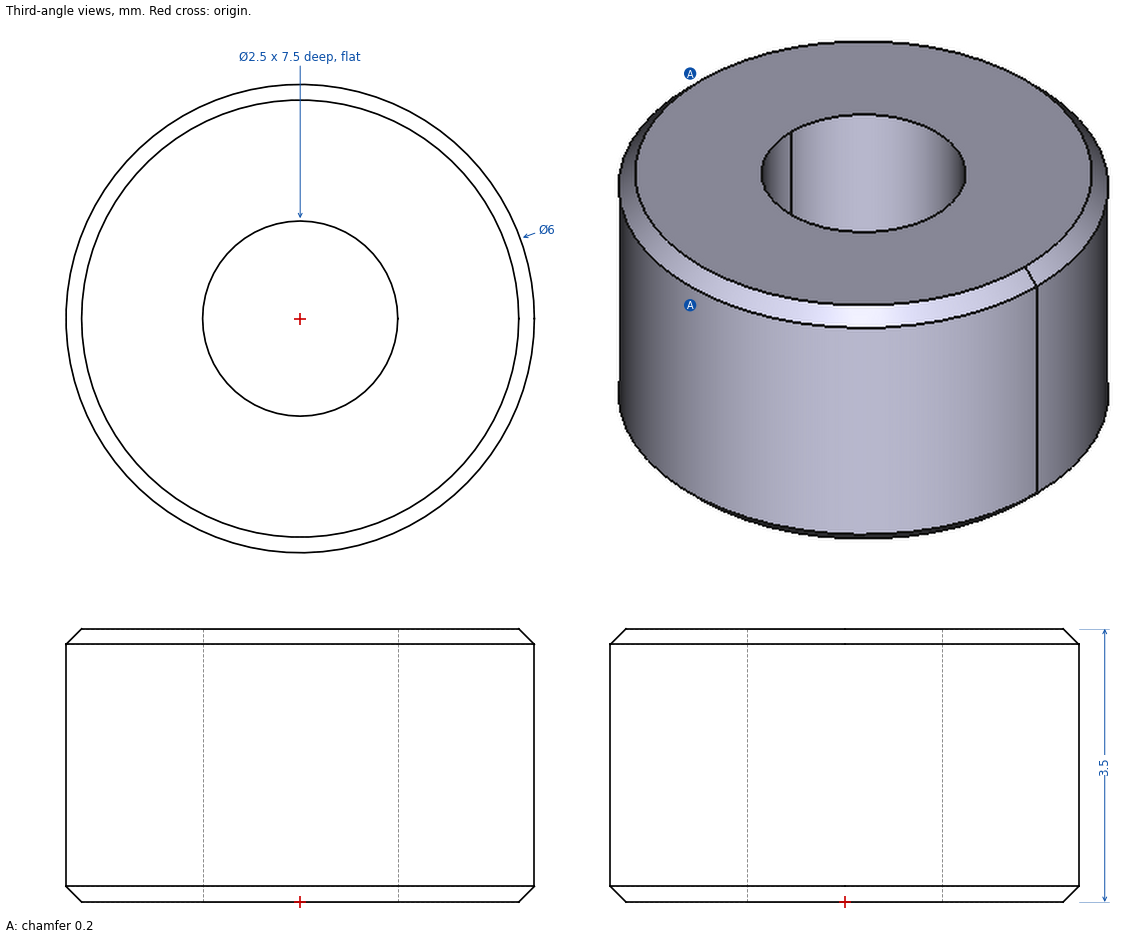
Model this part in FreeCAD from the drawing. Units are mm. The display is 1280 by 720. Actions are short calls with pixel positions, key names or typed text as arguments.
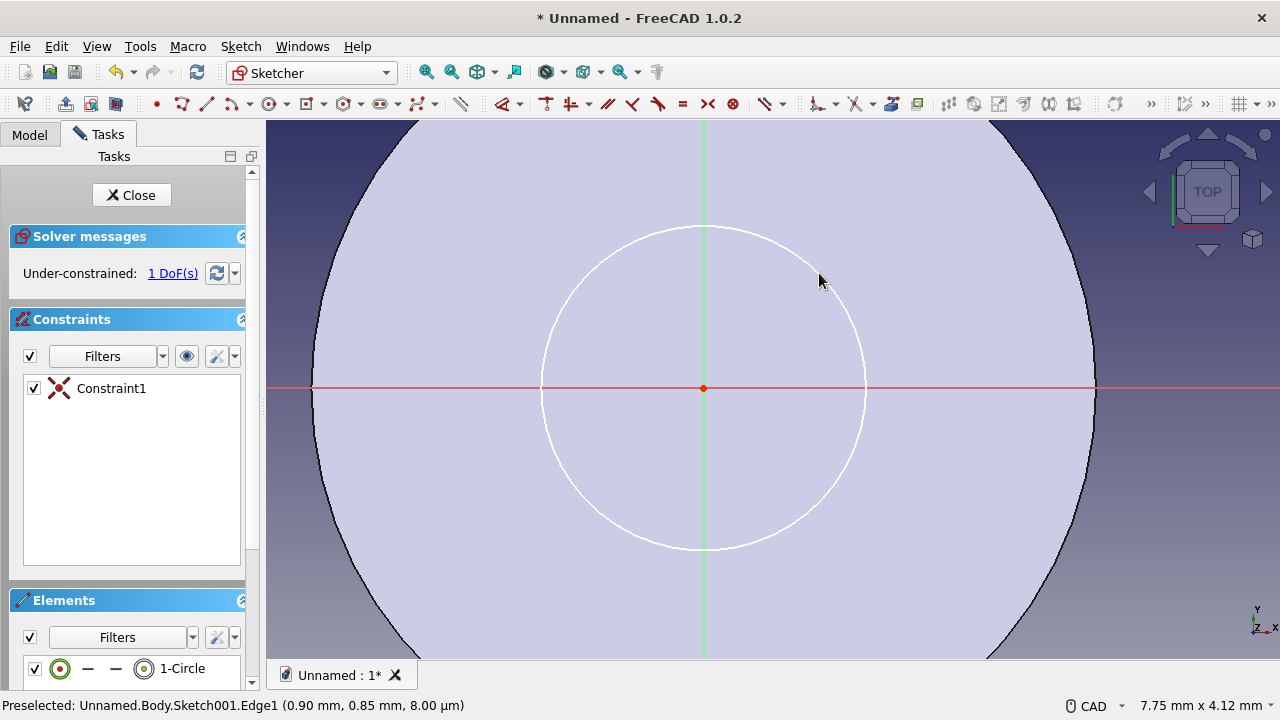
key(d)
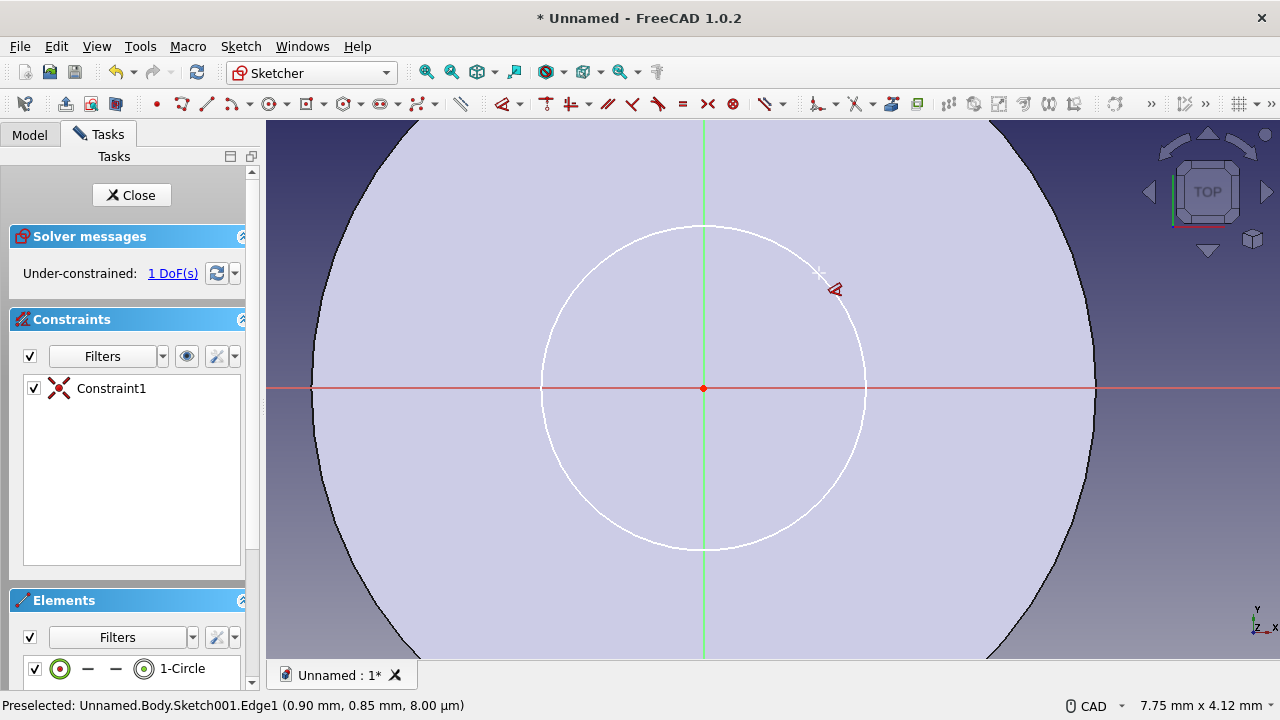
click(818, 273)
click(841, 250)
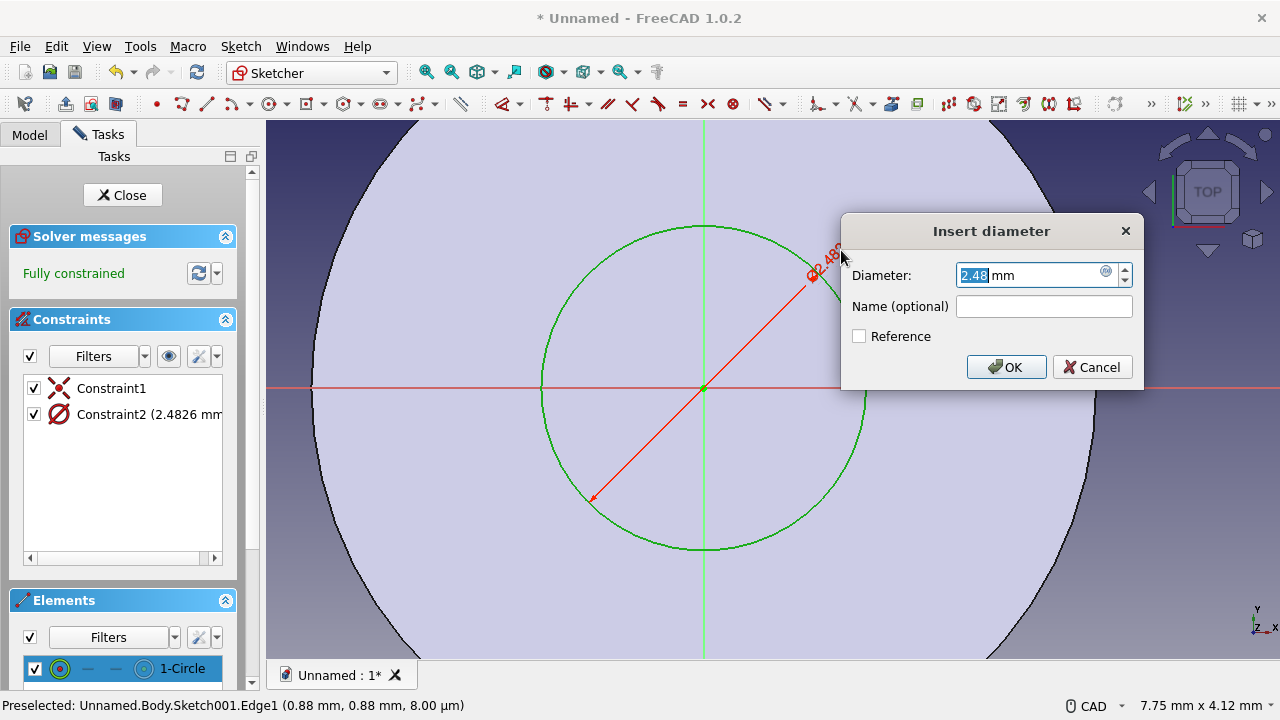
text(2.5)
key(Return)
key(Escape)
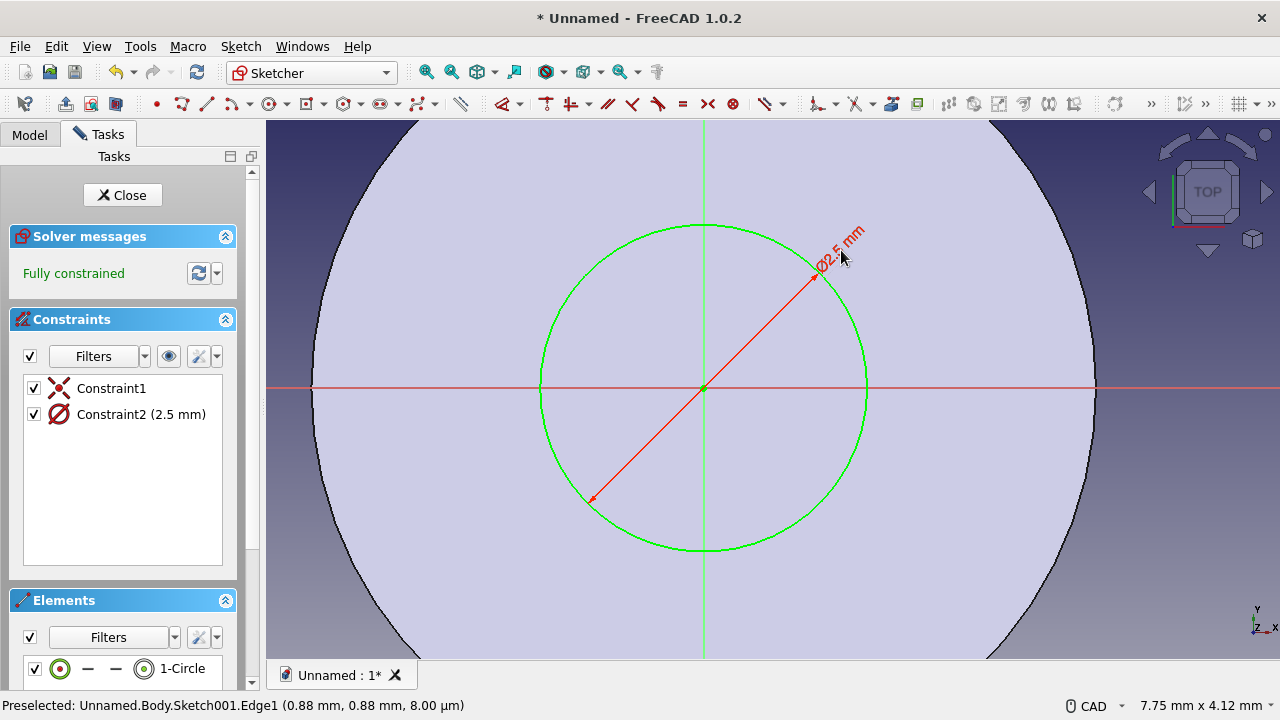
click(123, 195)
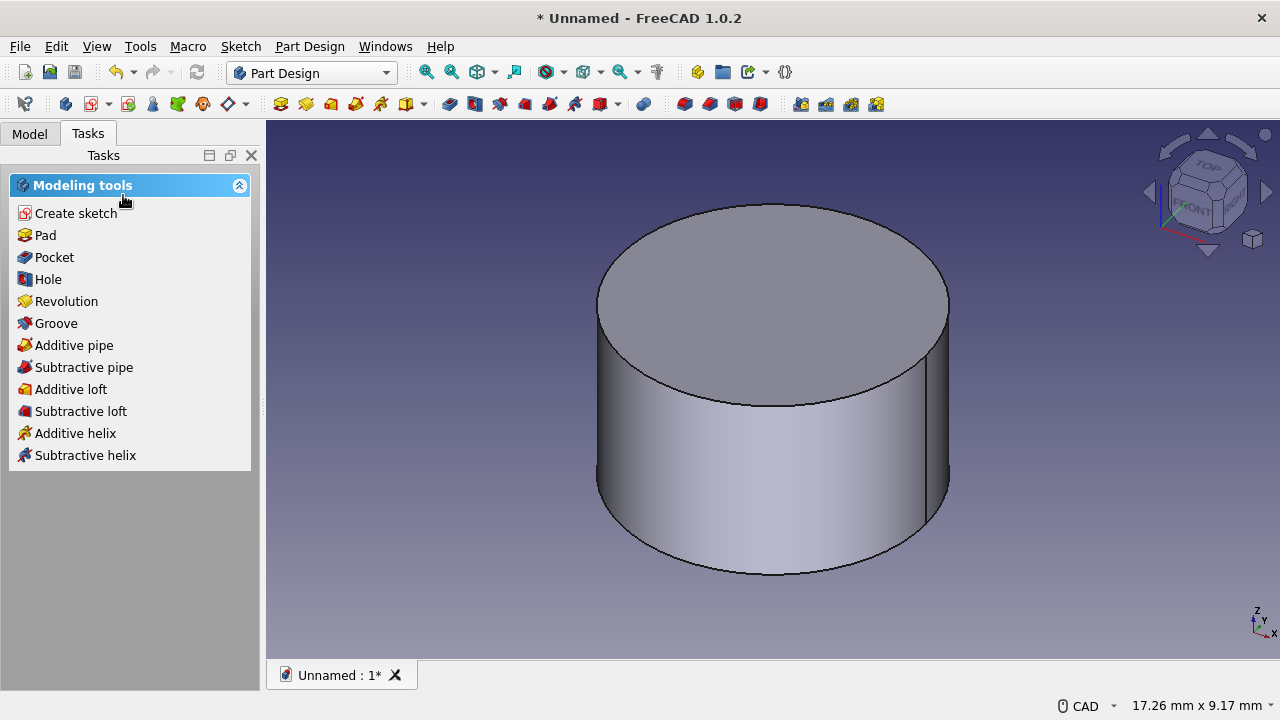
click(475, 104)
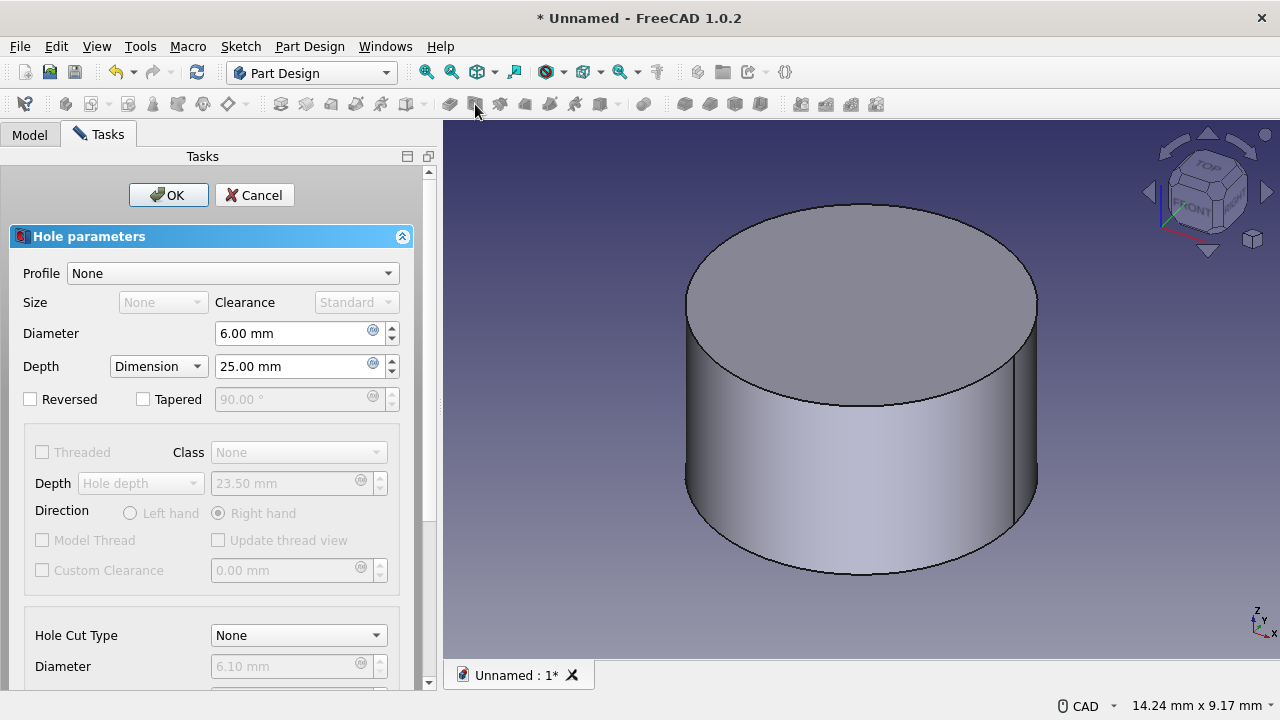
triple_click(300, 334)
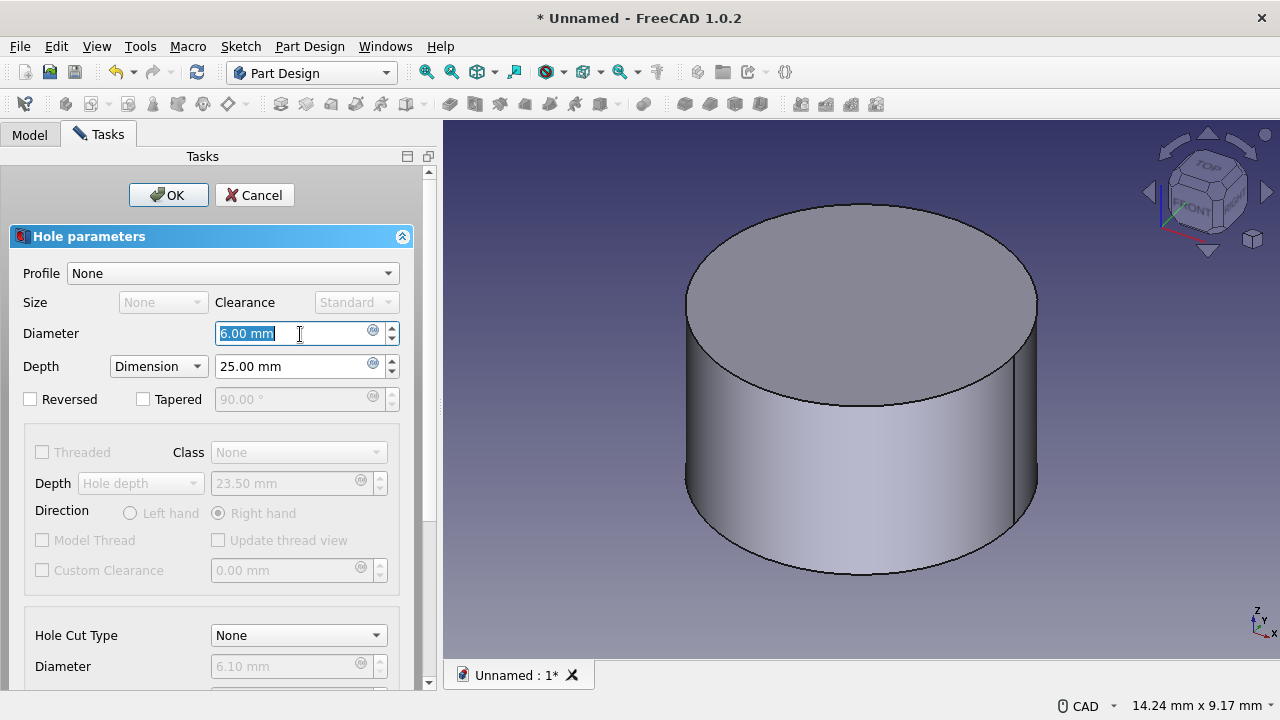
text(2.5)
key(Tab)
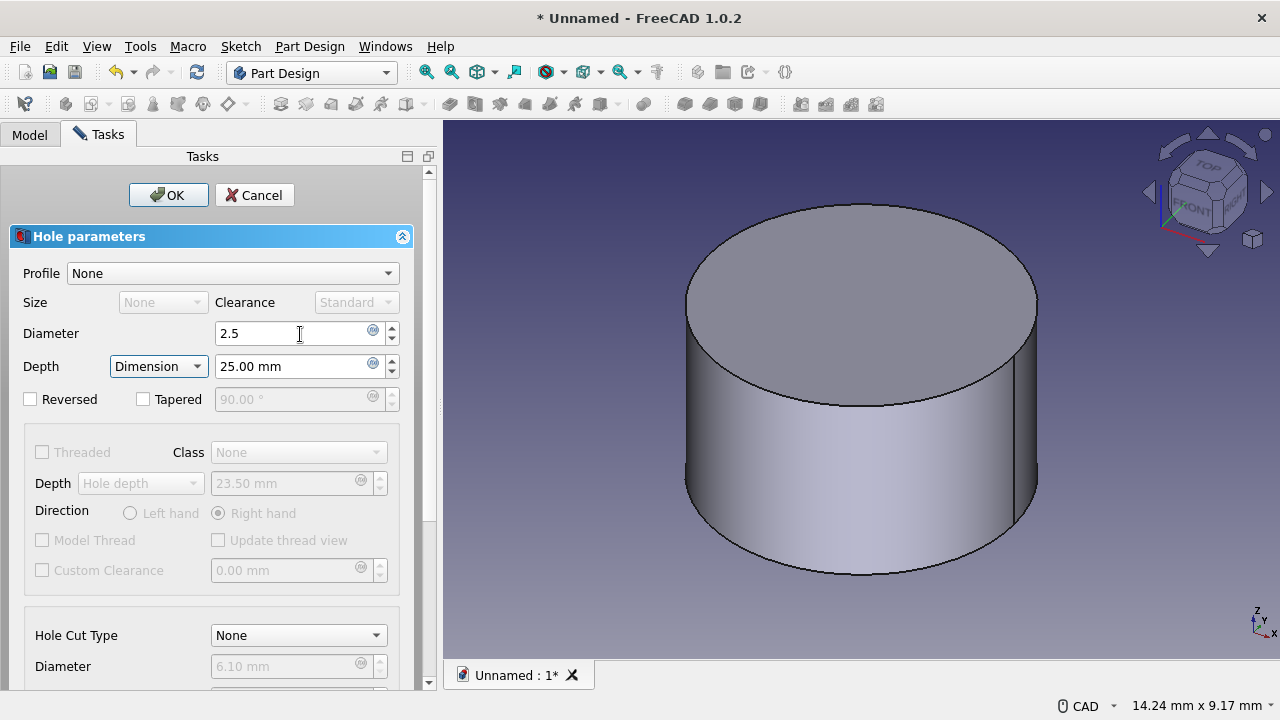
triple_click(300, 366)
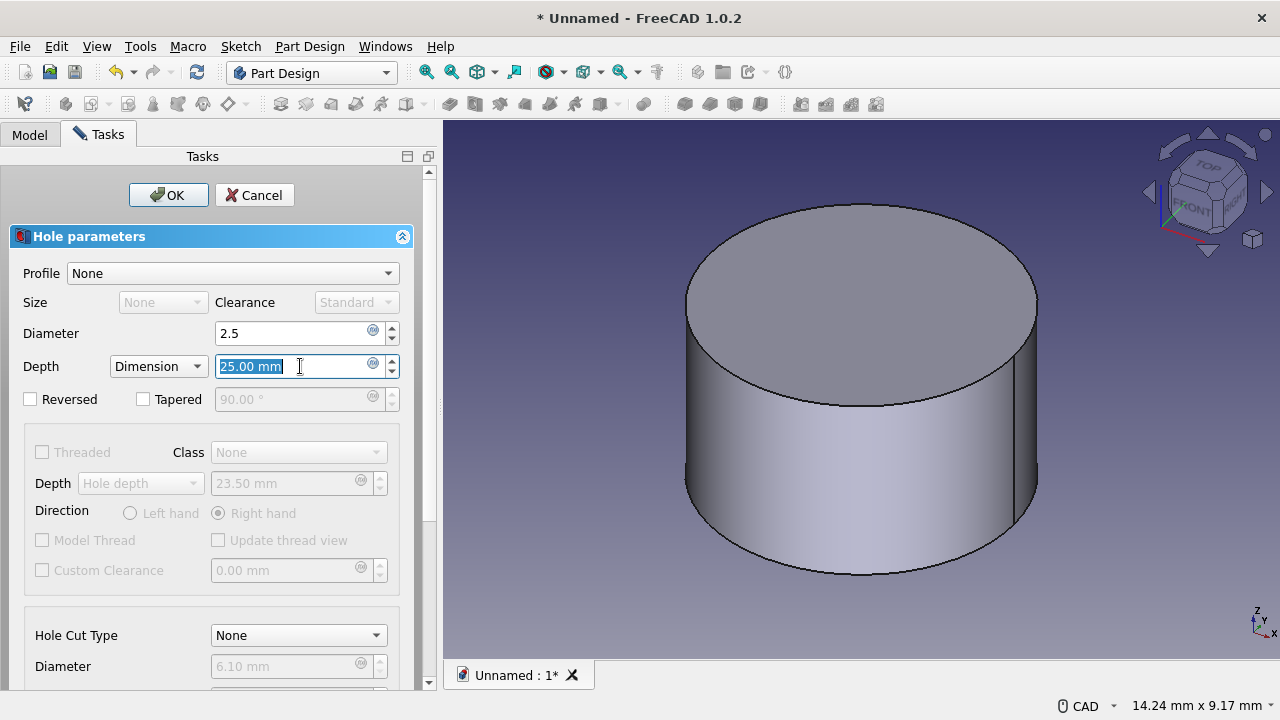
text(7.5)
key(Tab)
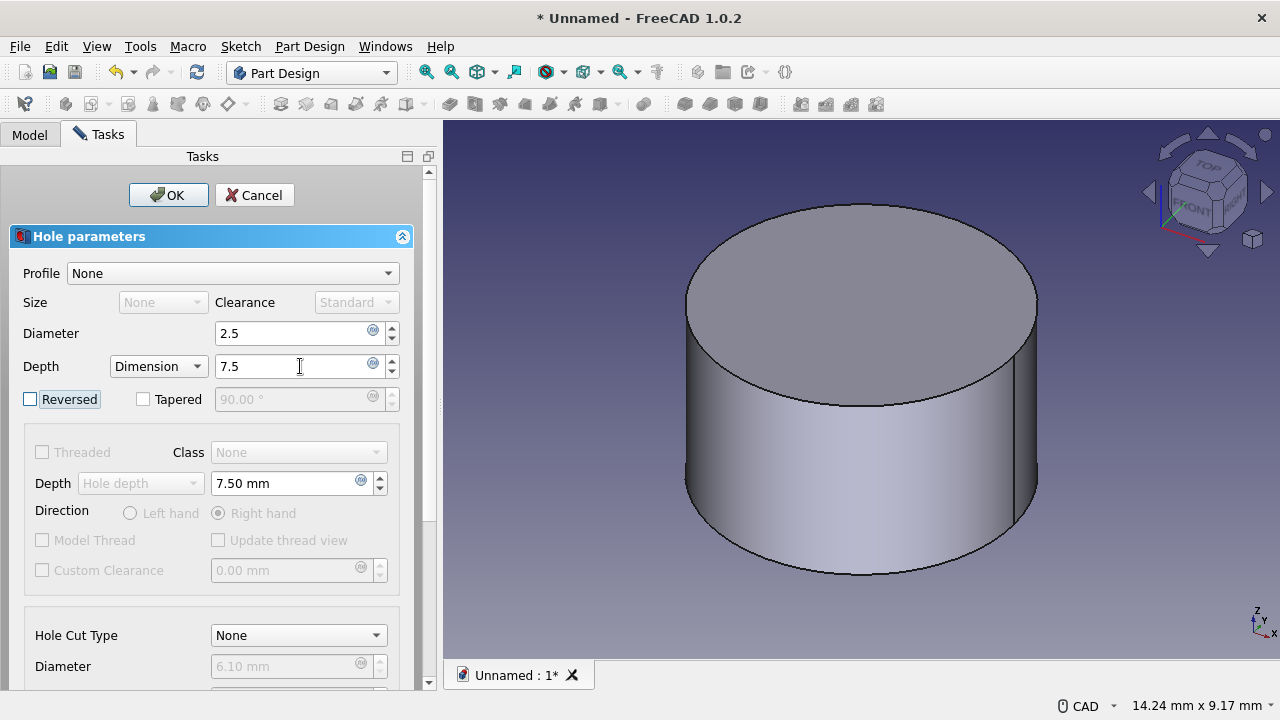
click(31, 399)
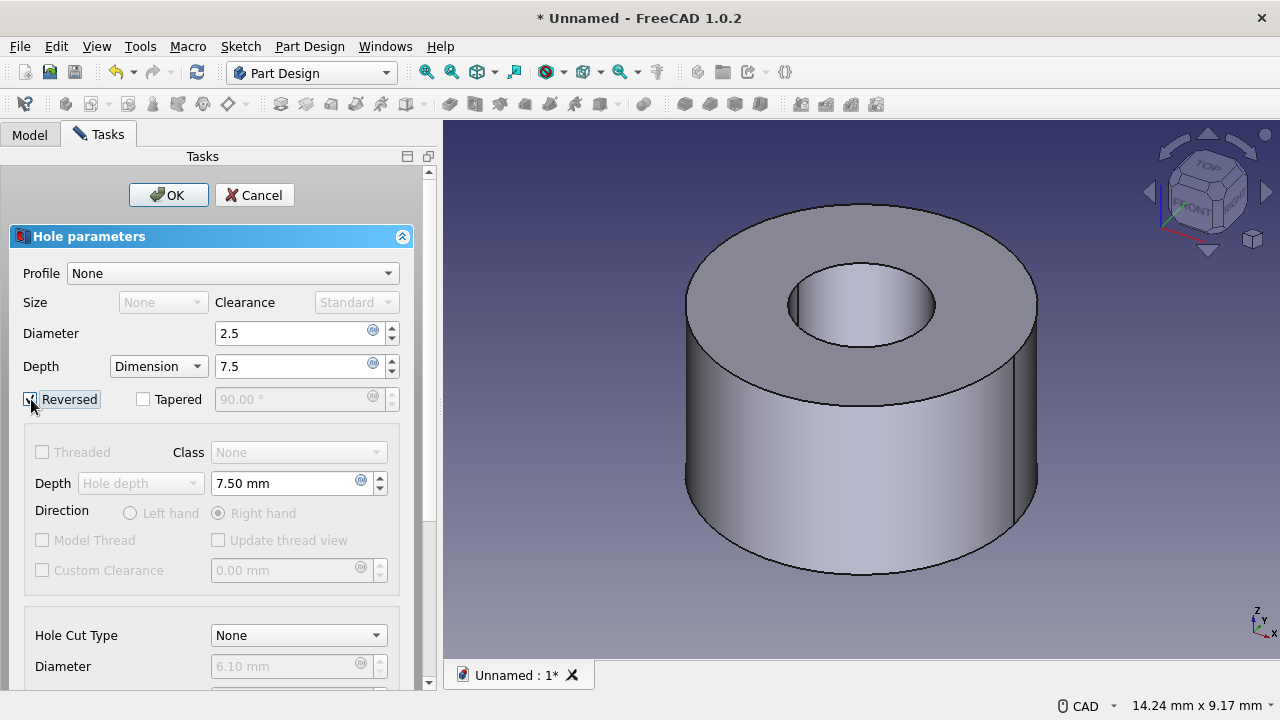
scroll(429, 428, down, 4)